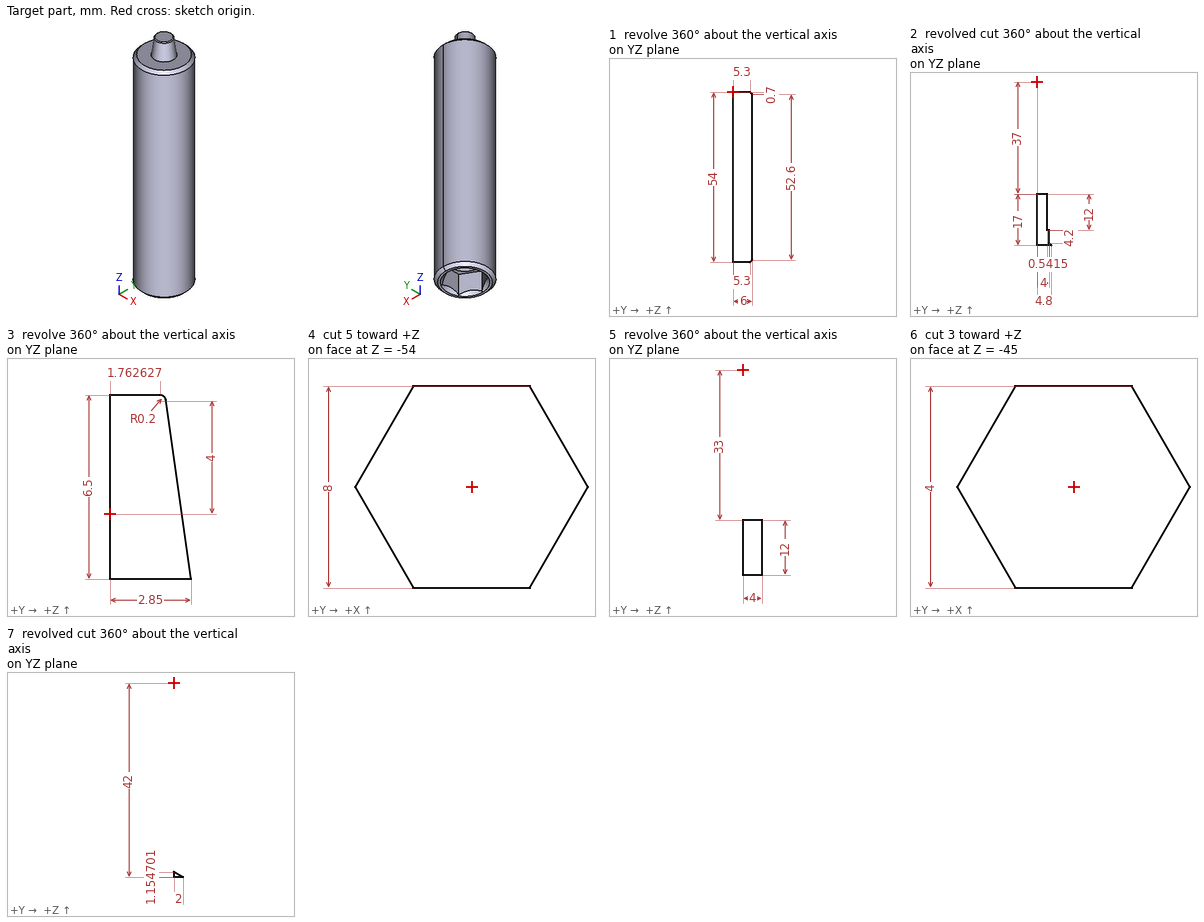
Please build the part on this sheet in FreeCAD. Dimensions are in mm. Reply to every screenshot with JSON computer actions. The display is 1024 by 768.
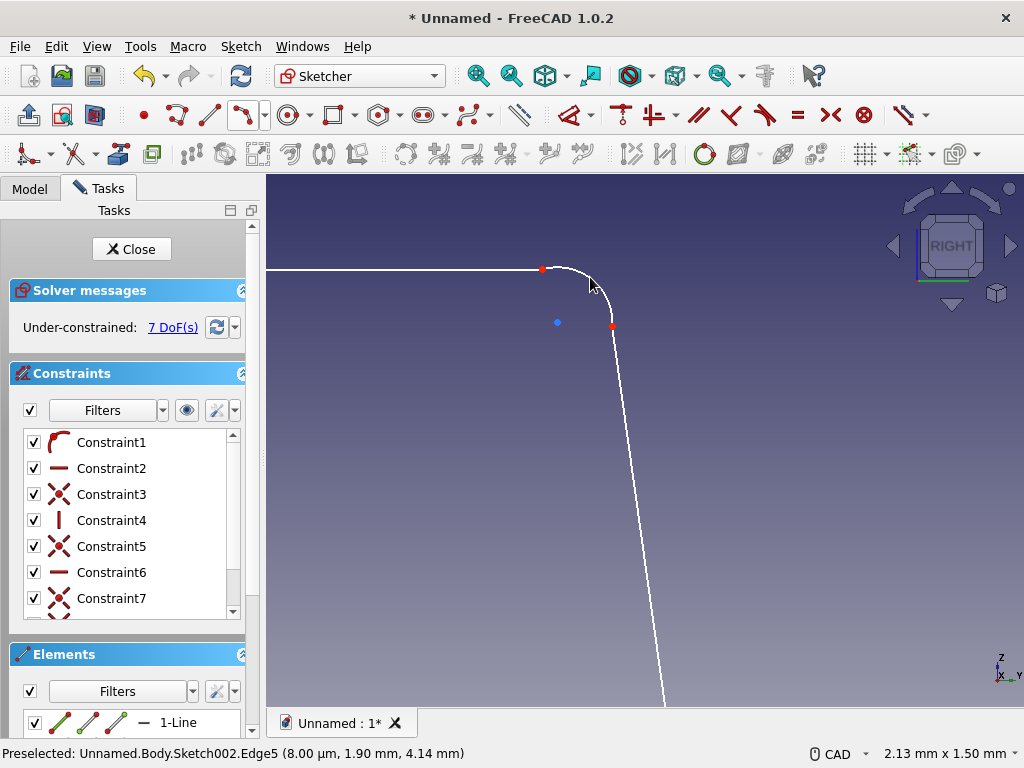
{"action": "scroll", "coordinate": [600, 288], "scroll_direction": "down", "scroll_amount": 10}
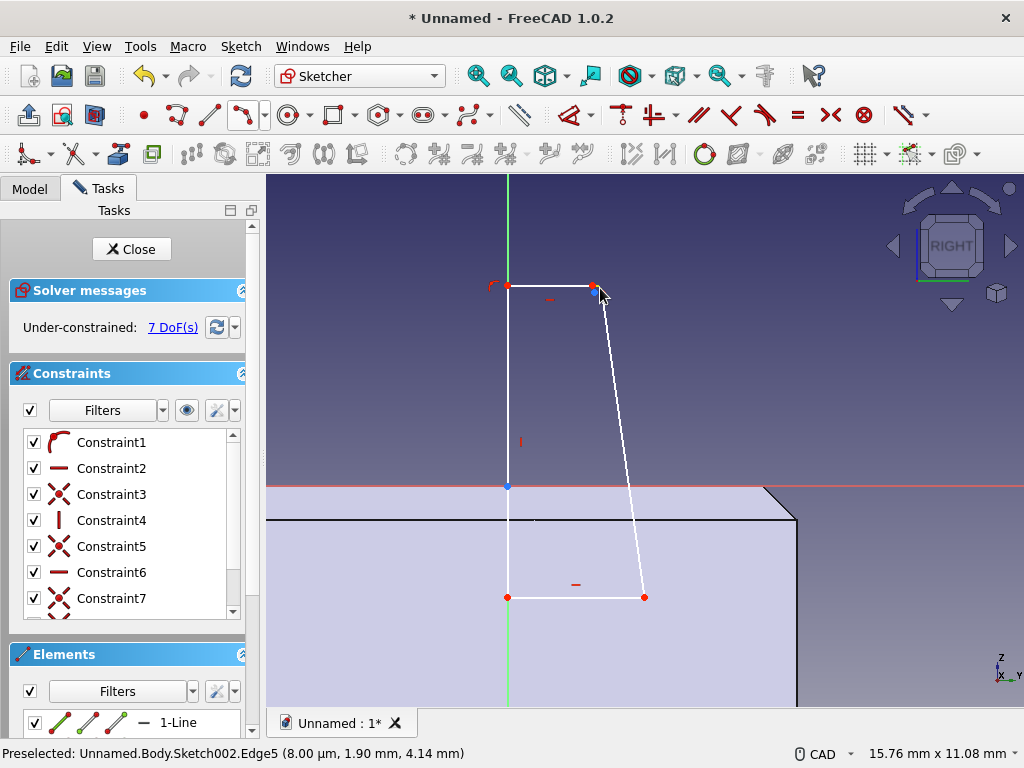
{"action": "left_click", "coordinate": [567, 286]}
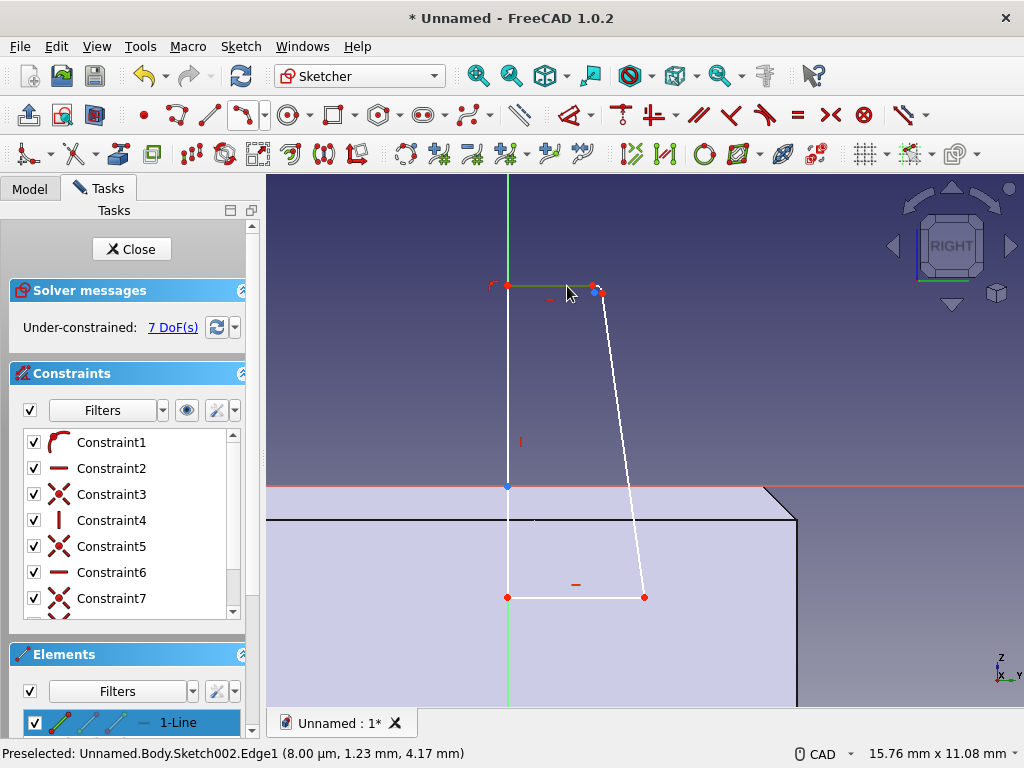
{"action": "scroll", "coordinate": [599, 287], "scroll_direction": "up", "scroll_amount": 4}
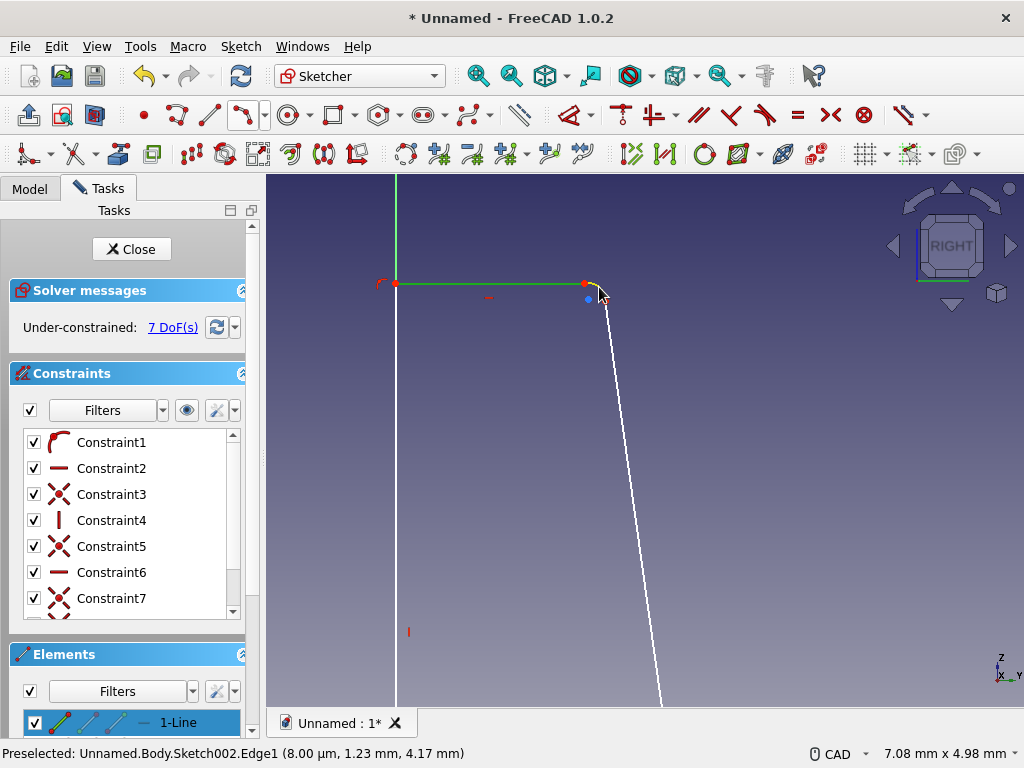
{"action": "left_click", "coordinate": [599, 287]}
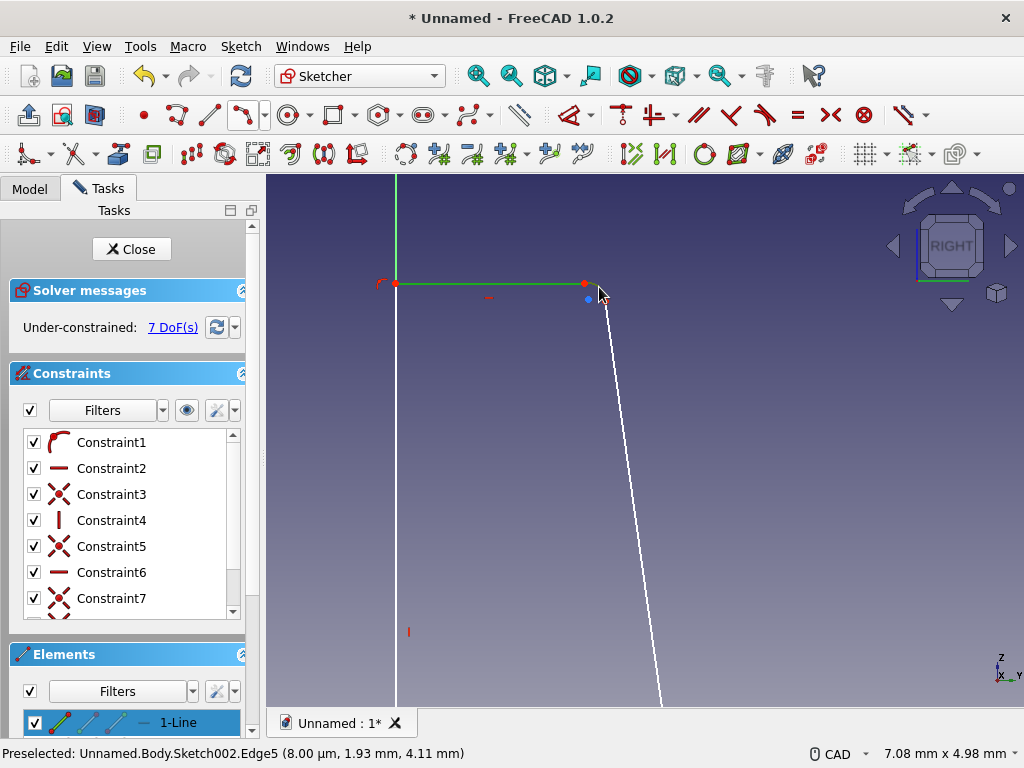
{"action": "left_click", "coordinate": [765, 116]}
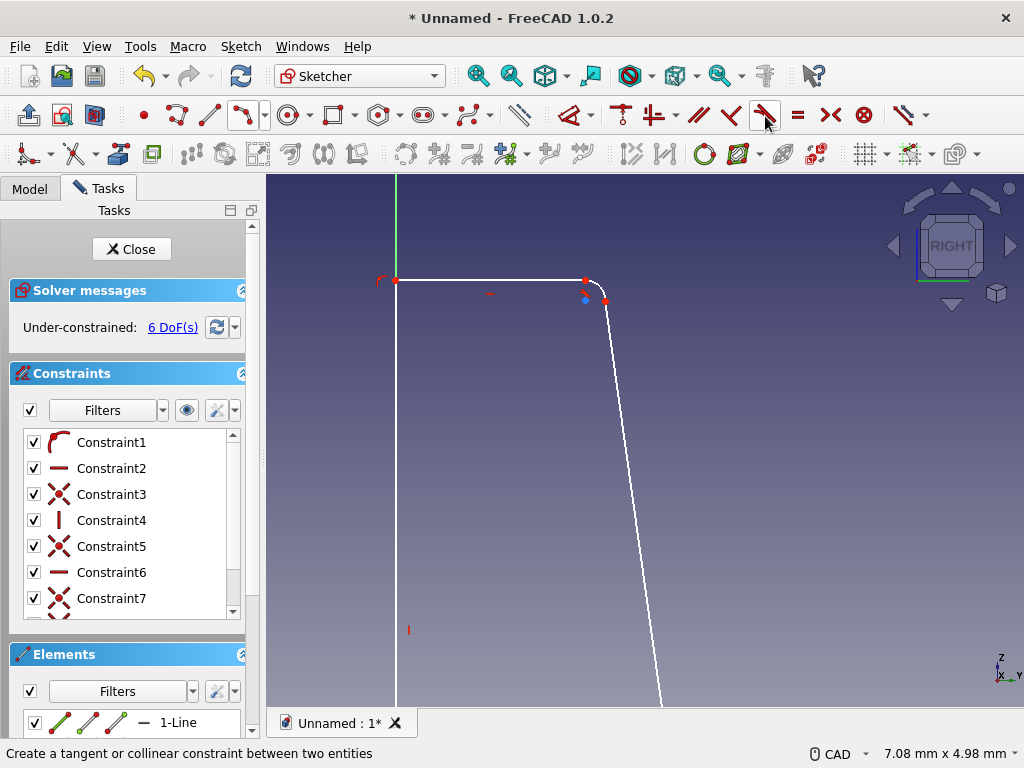
{"action": "left_click", "coordinate": [634, 505]}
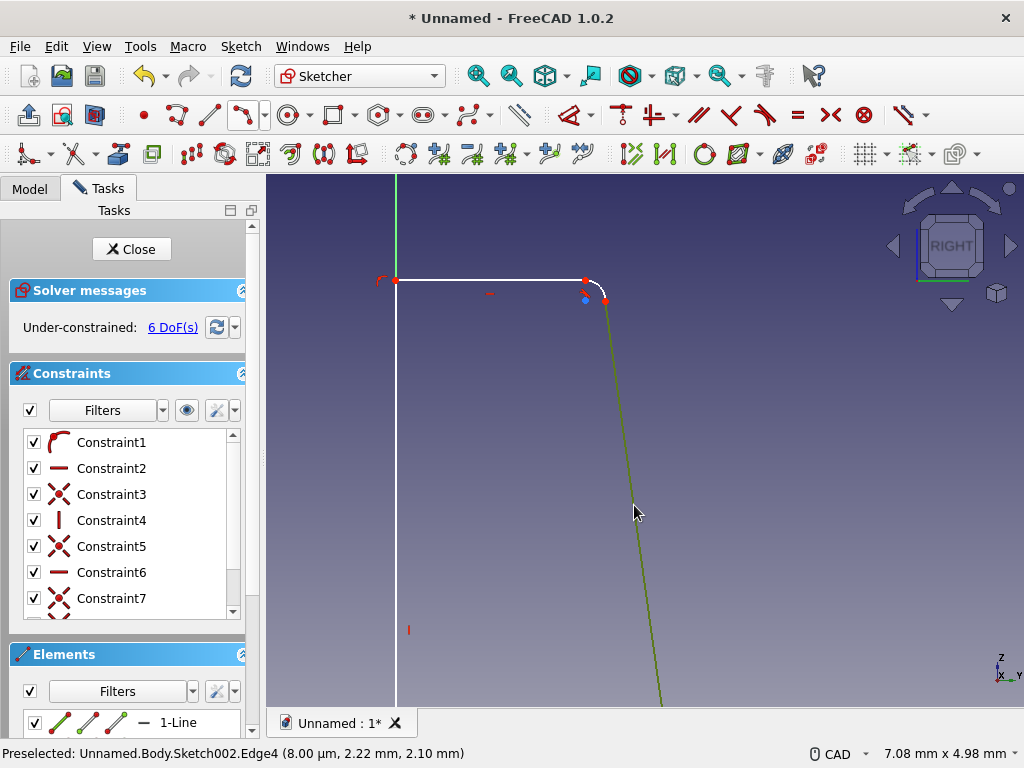
{"action": "scroll", "coordinate": [604, 292], "scroll_direction": "up", "scroll_amount": 2}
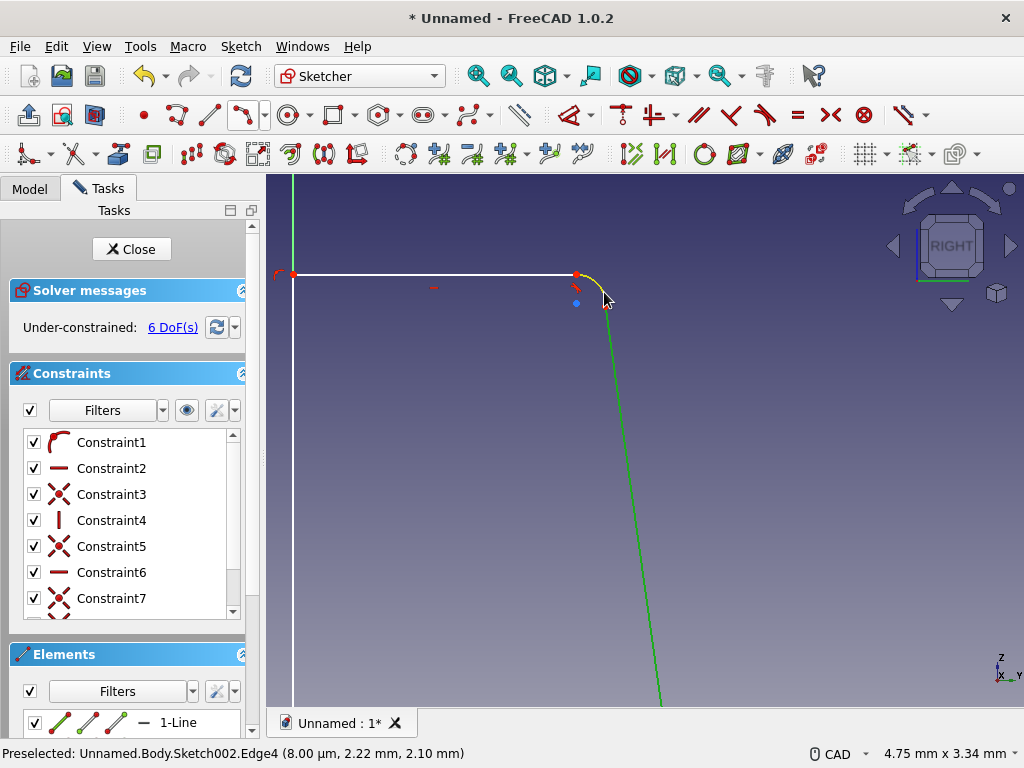
{"action": "left_click", "coordinate": [603, 292]}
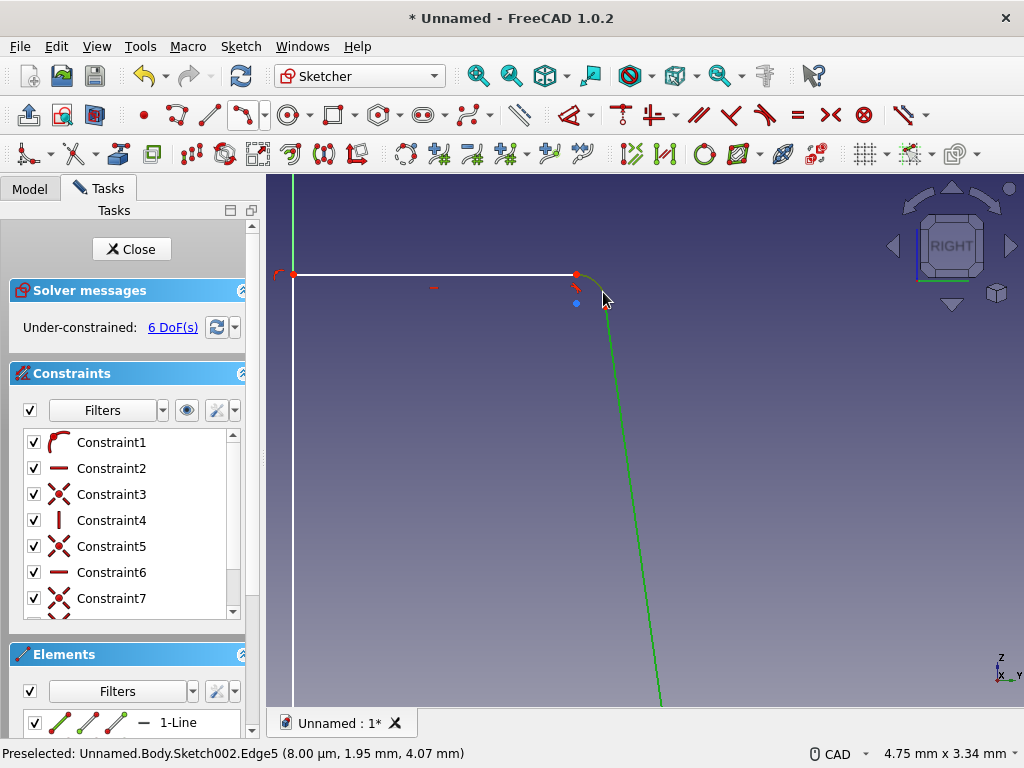
{"action": "left_click", "coordinate": [765, 116]}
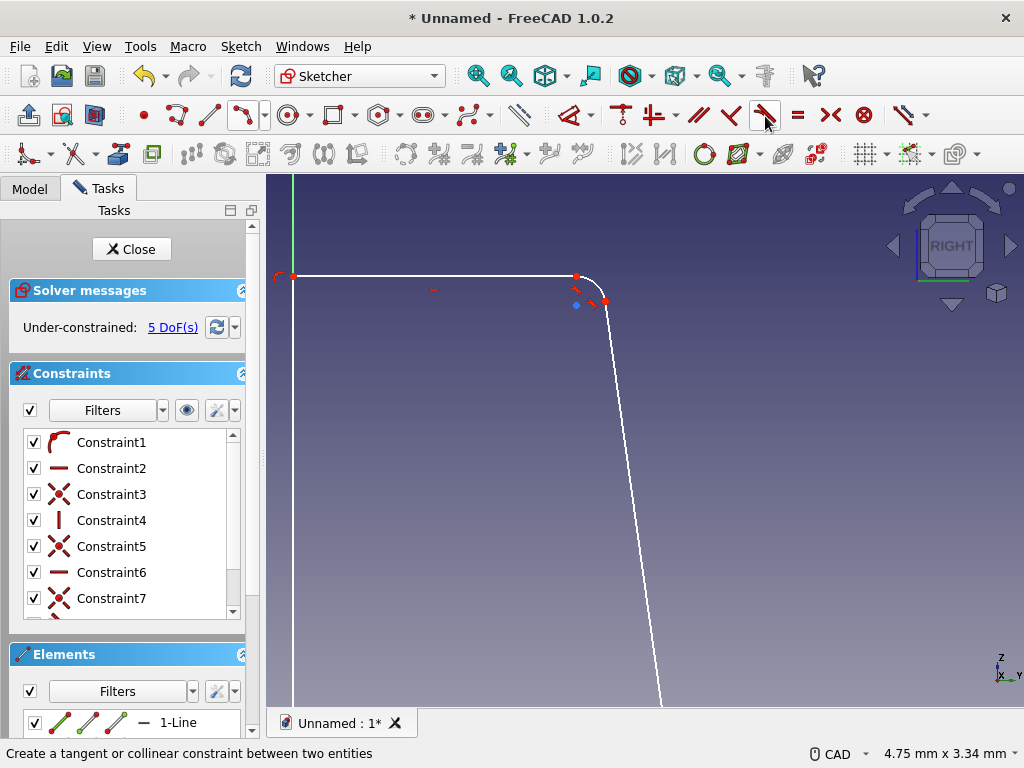
{"action": "left_click", "coordinate": [568, 116]}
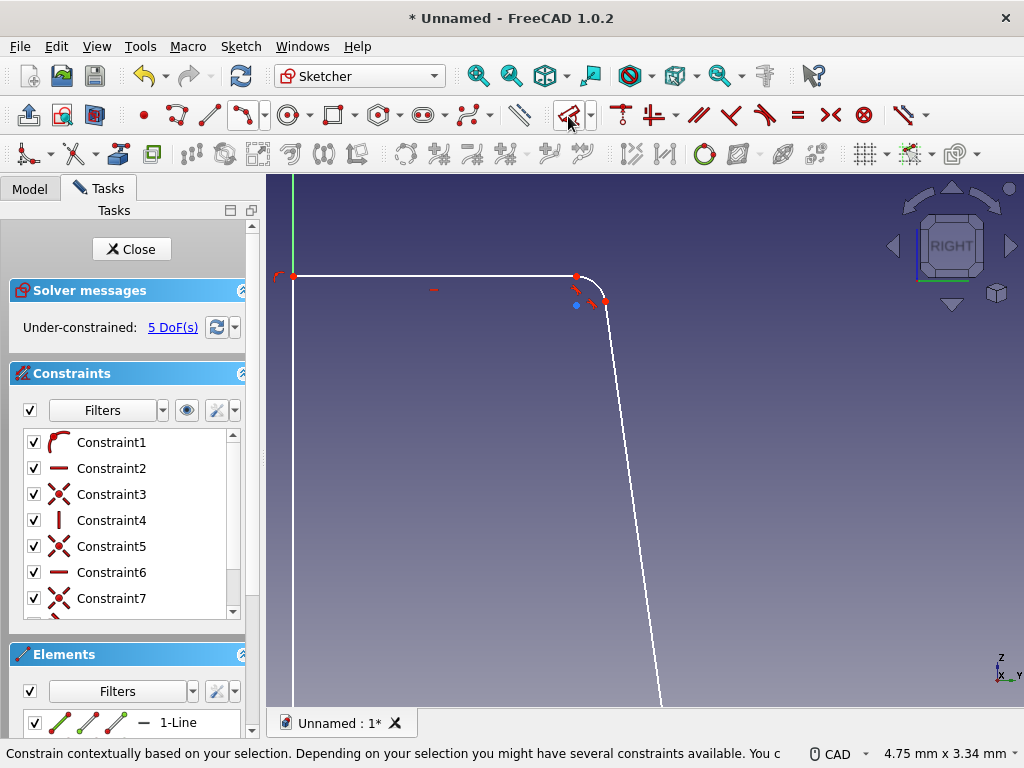
{"action": "scroll", "coordinate": [601, 290], "scroll_direction": "up", "scroll_amount": 2}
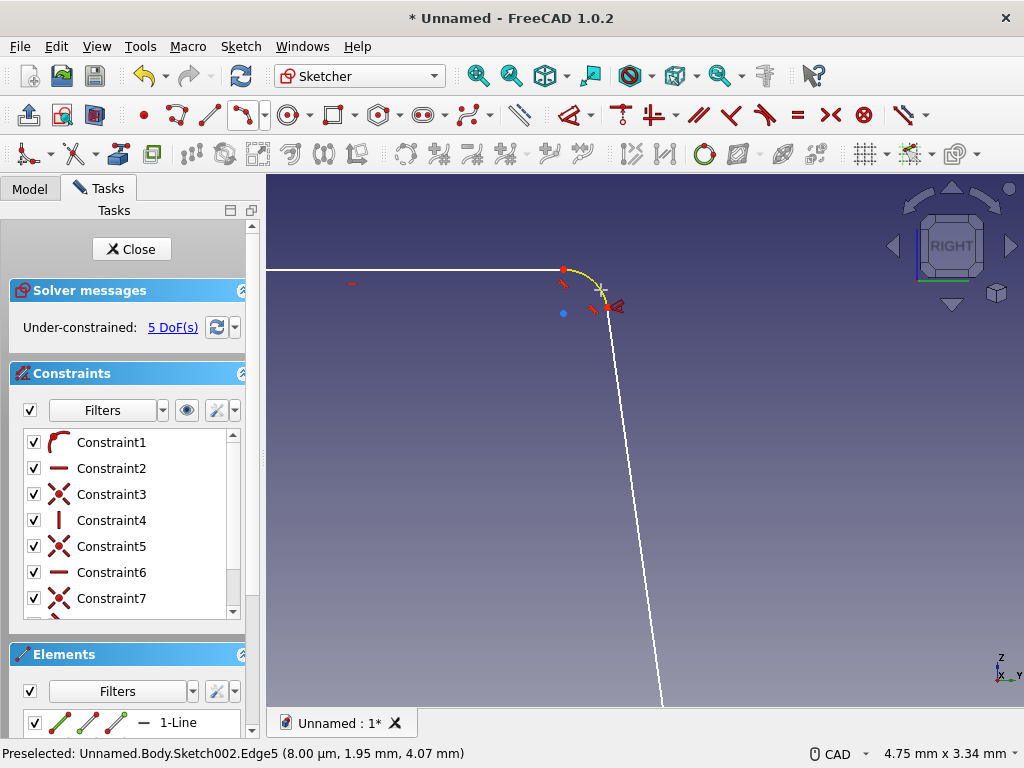
{"action": "left_click", "coordinate": [601, 290]}
{"action": "left_click", "coordinate": [628, 273]}